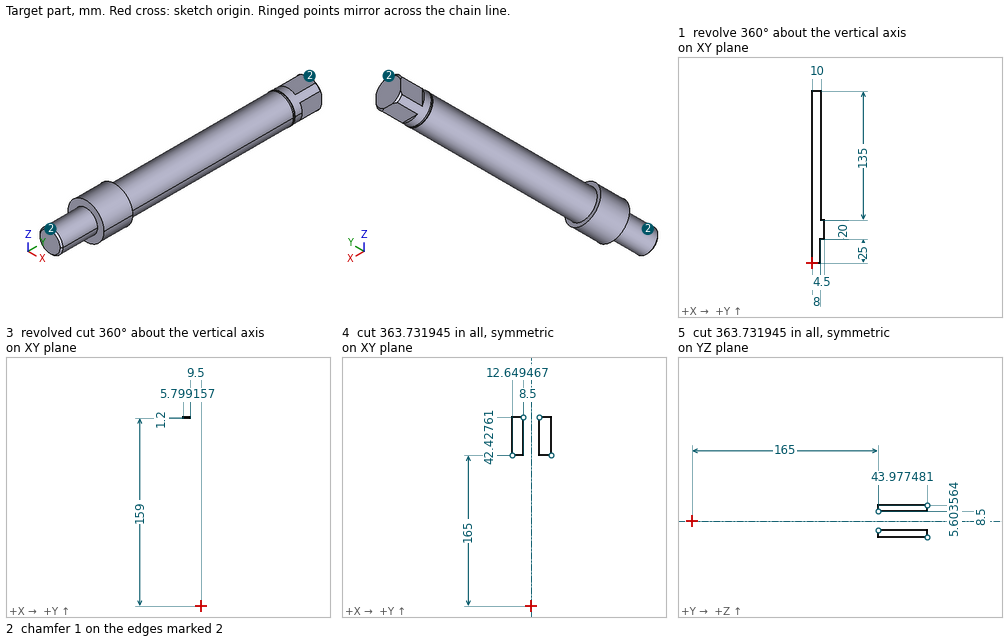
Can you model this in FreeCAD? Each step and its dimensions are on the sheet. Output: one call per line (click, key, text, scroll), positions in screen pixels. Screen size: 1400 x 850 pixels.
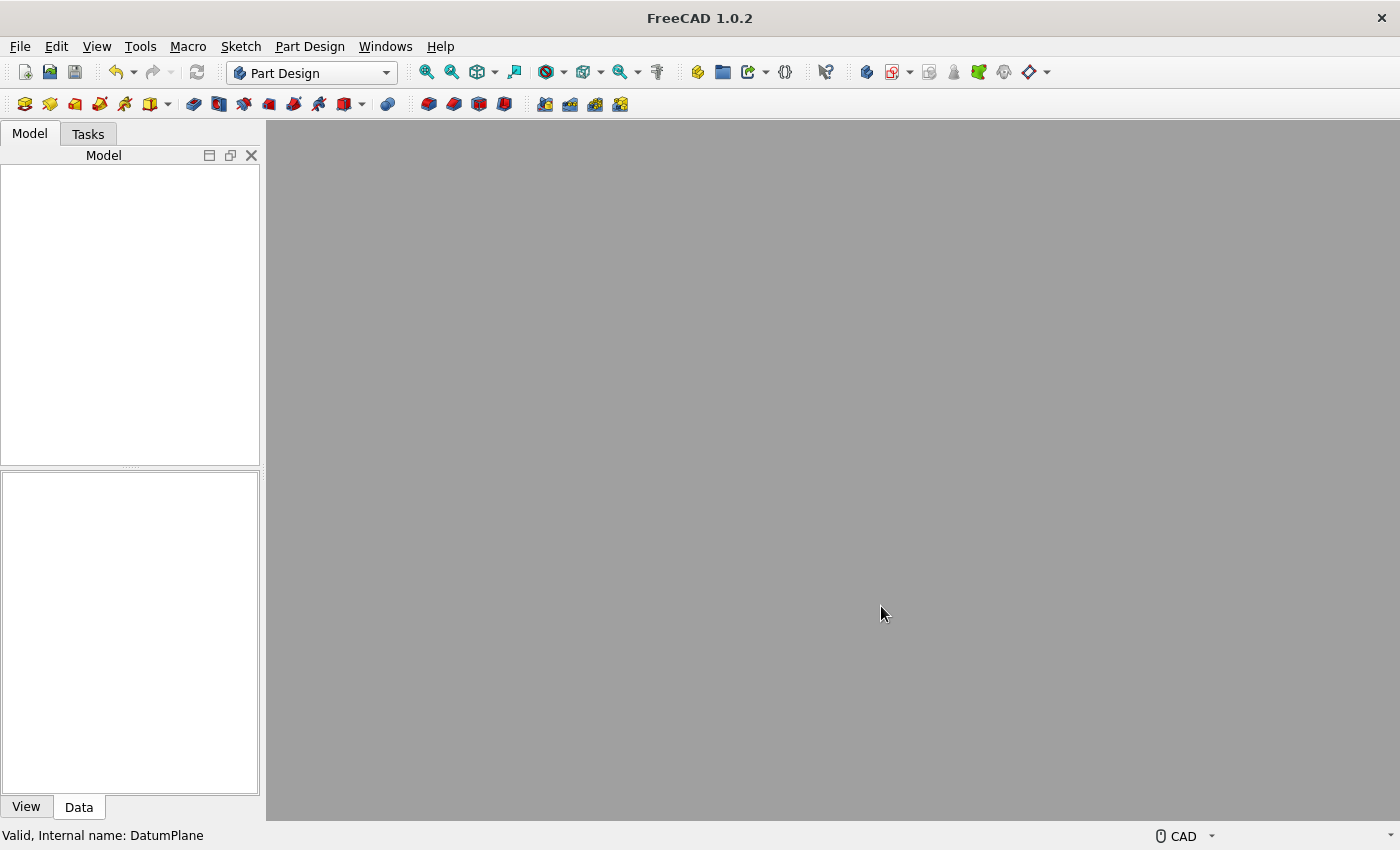
key(ctrl+n)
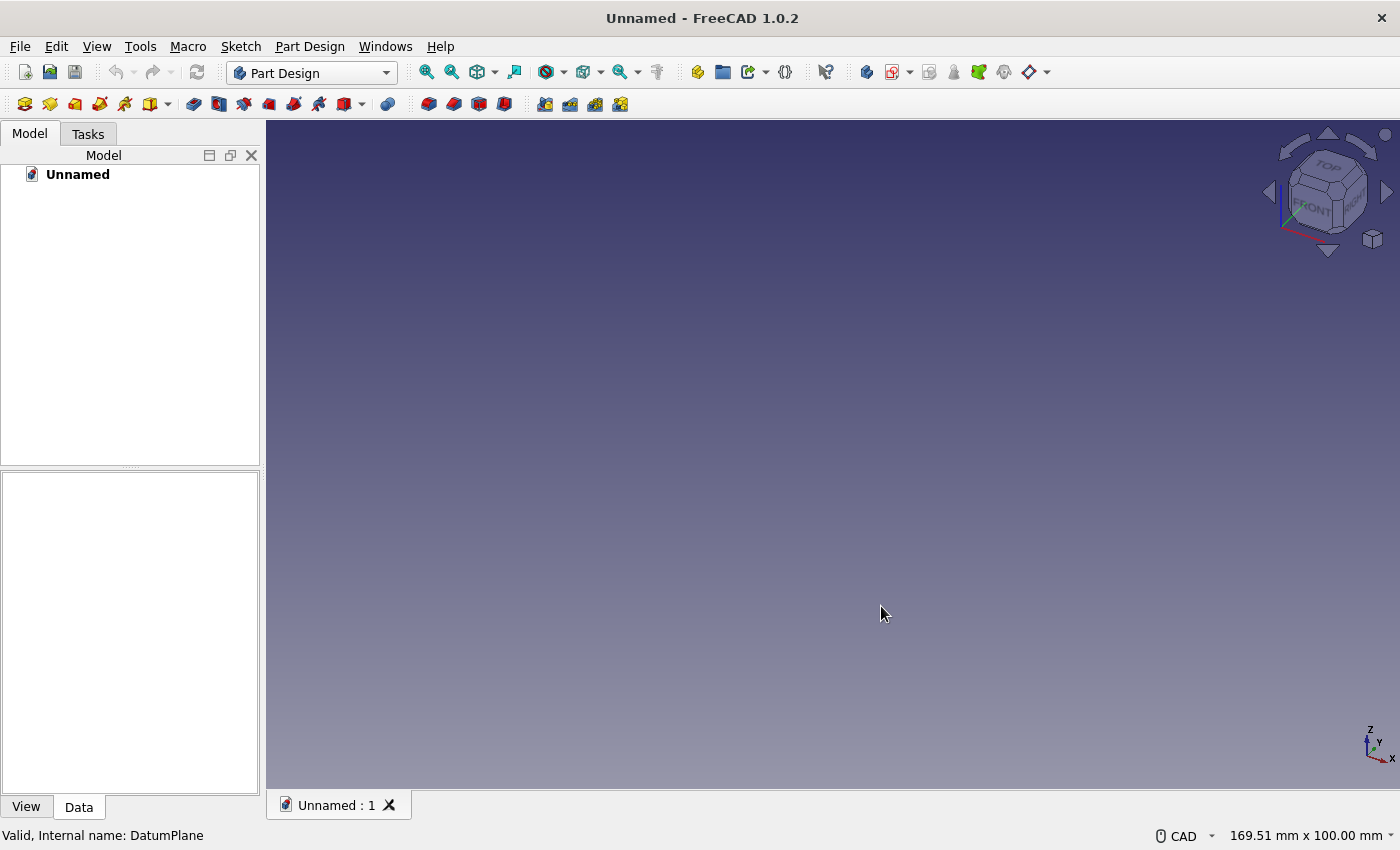
click(892, 72)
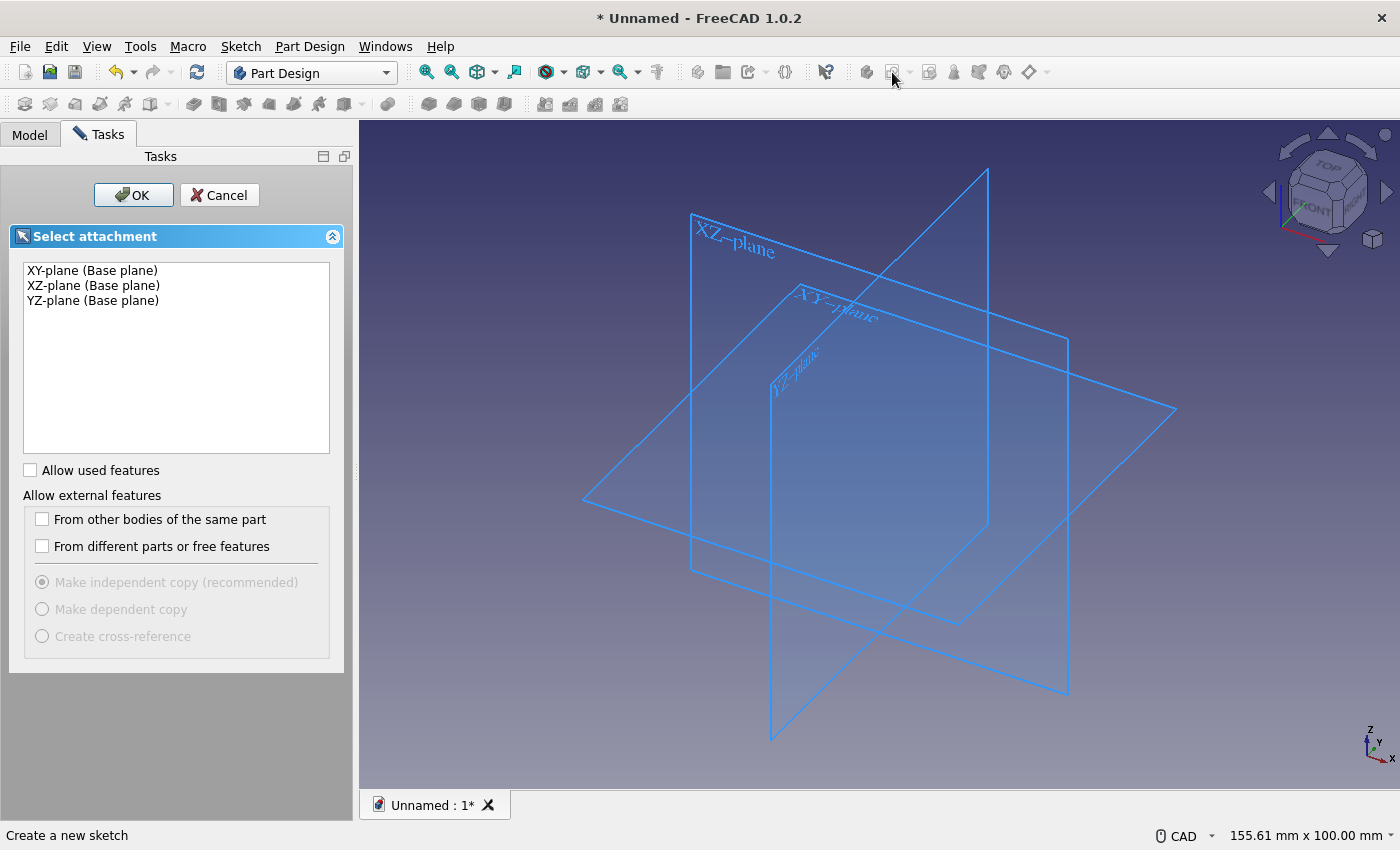
click(84, 270)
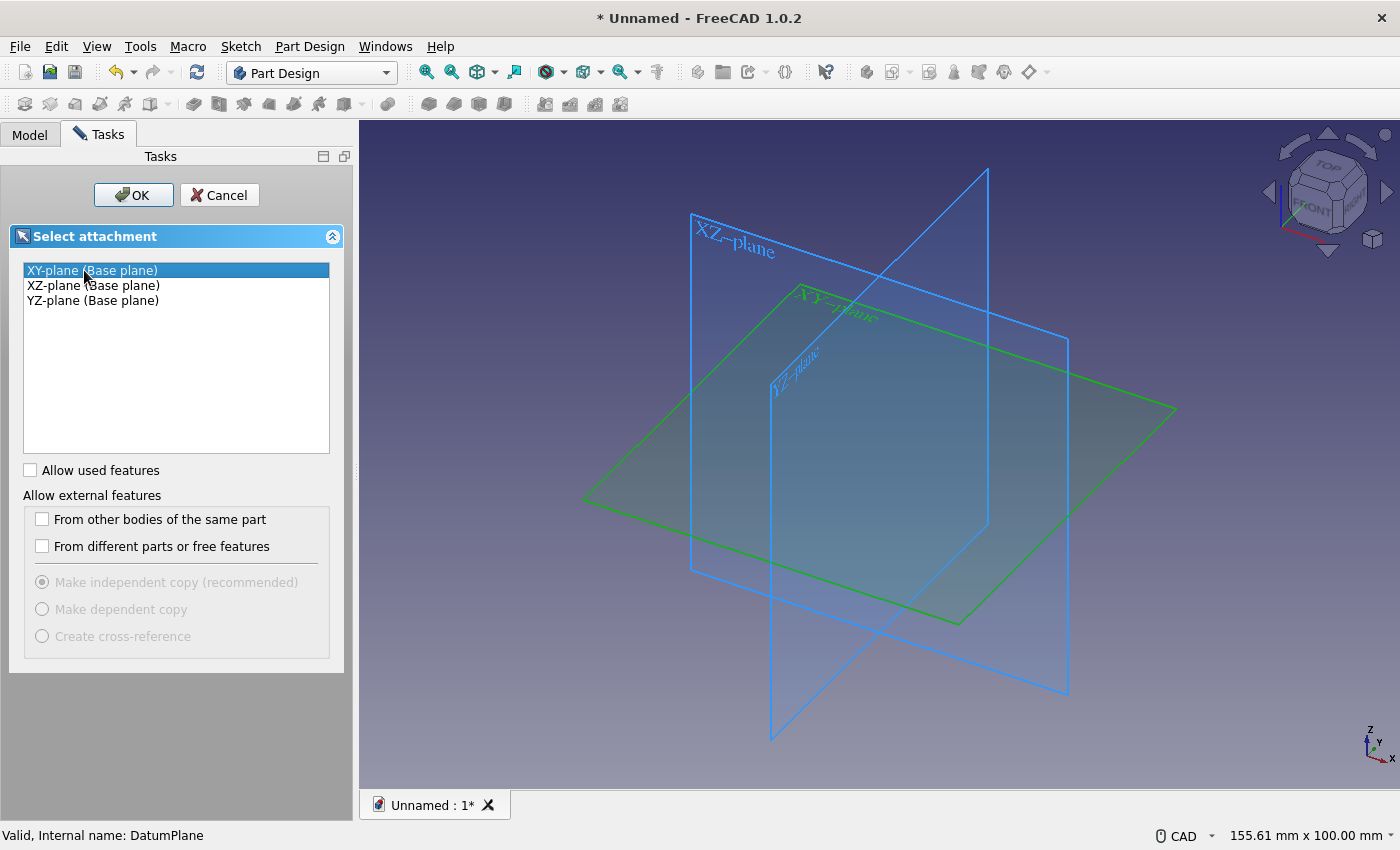
click(134, 195)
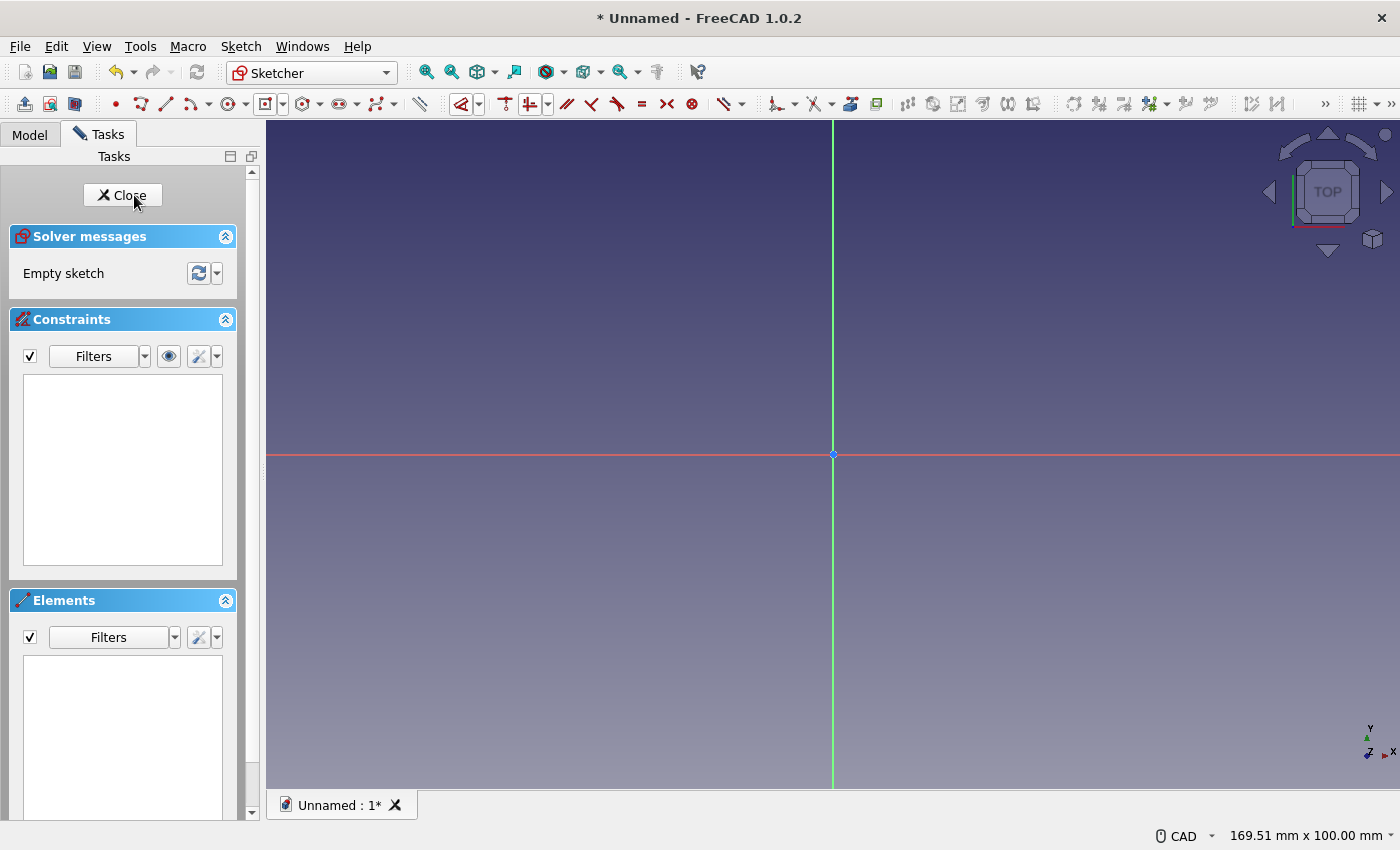
scroll(700, 761, down, 5)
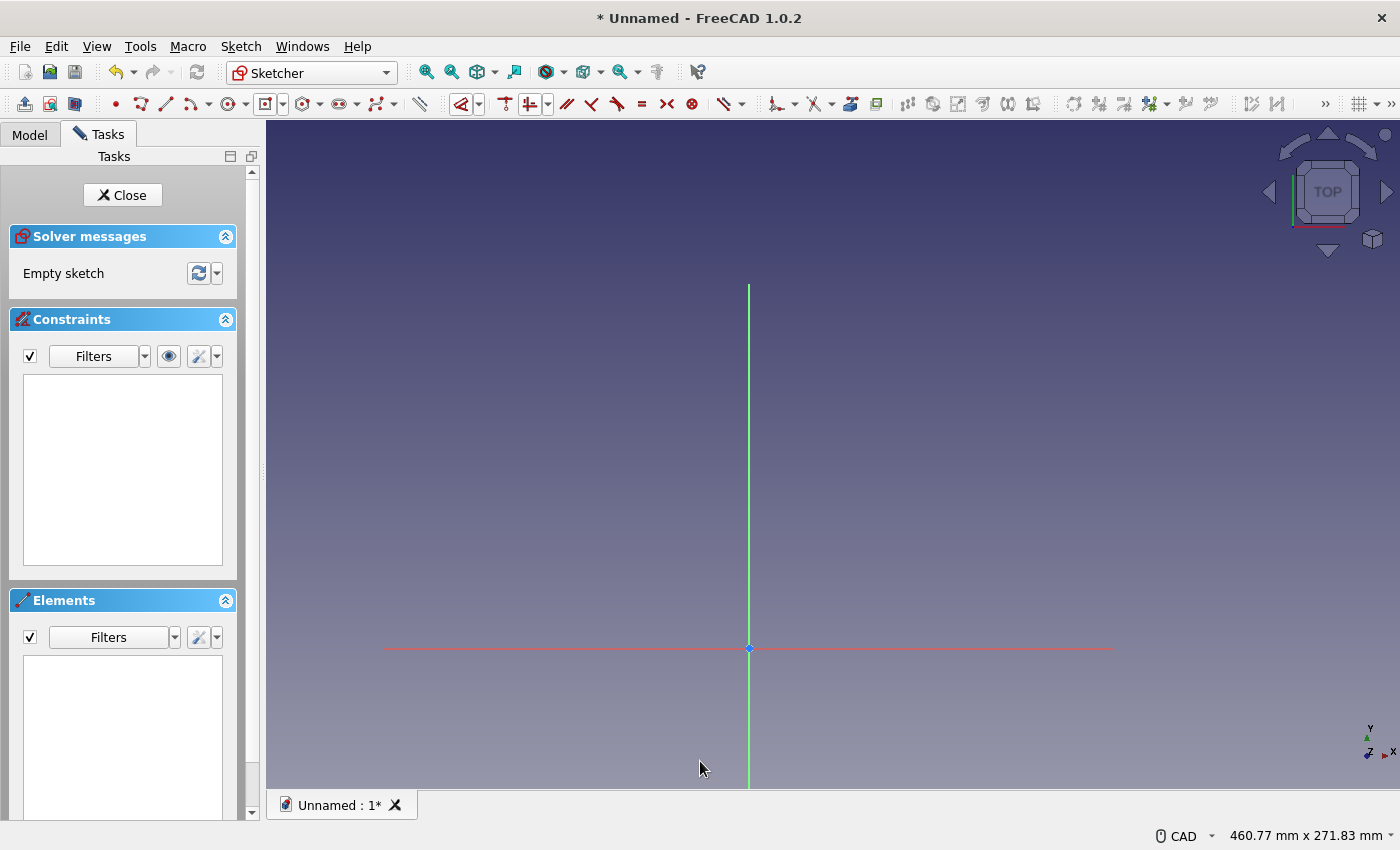
key(g)
key(m)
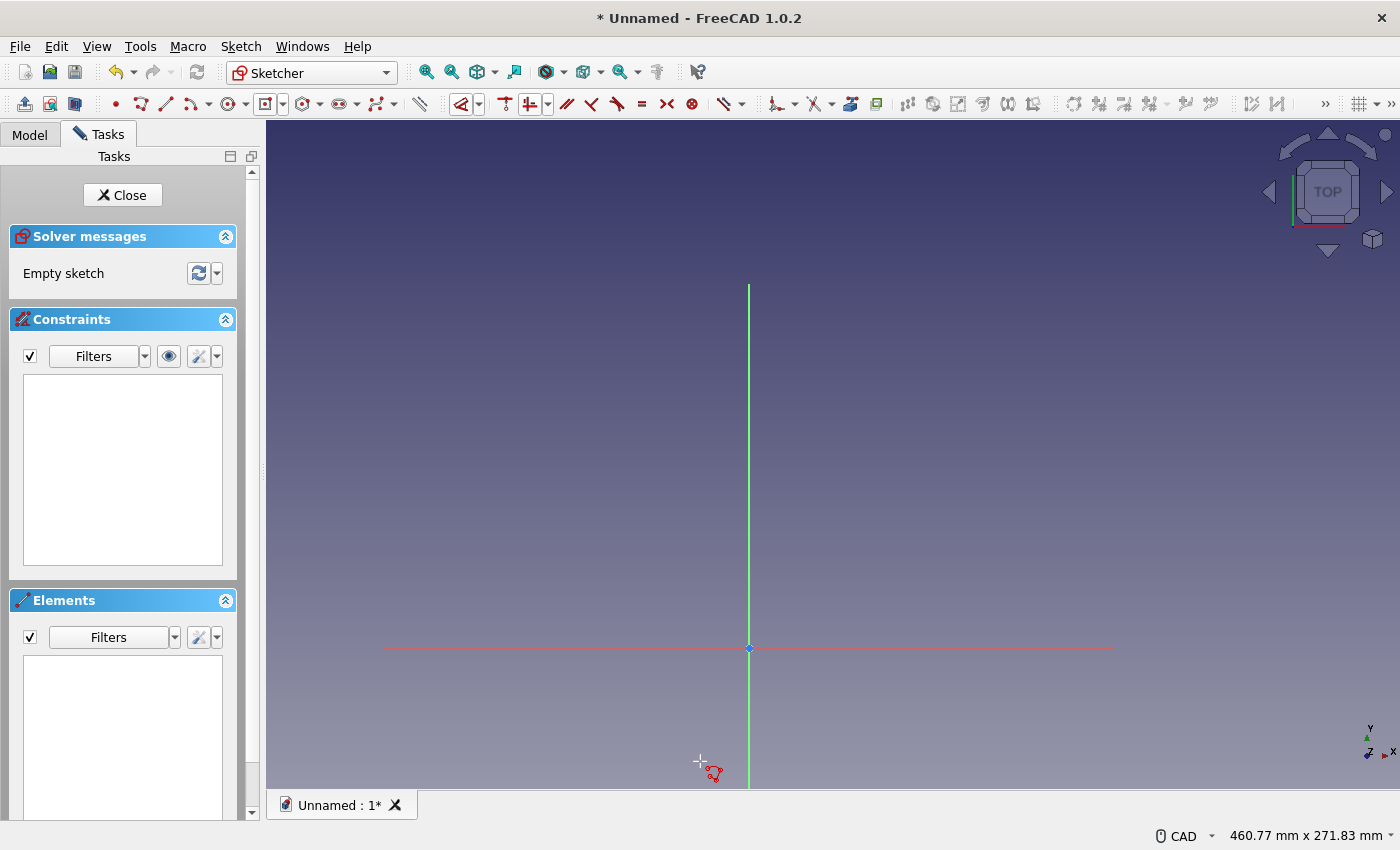
click(749, 649)
click(769, 640)
click(769, 587)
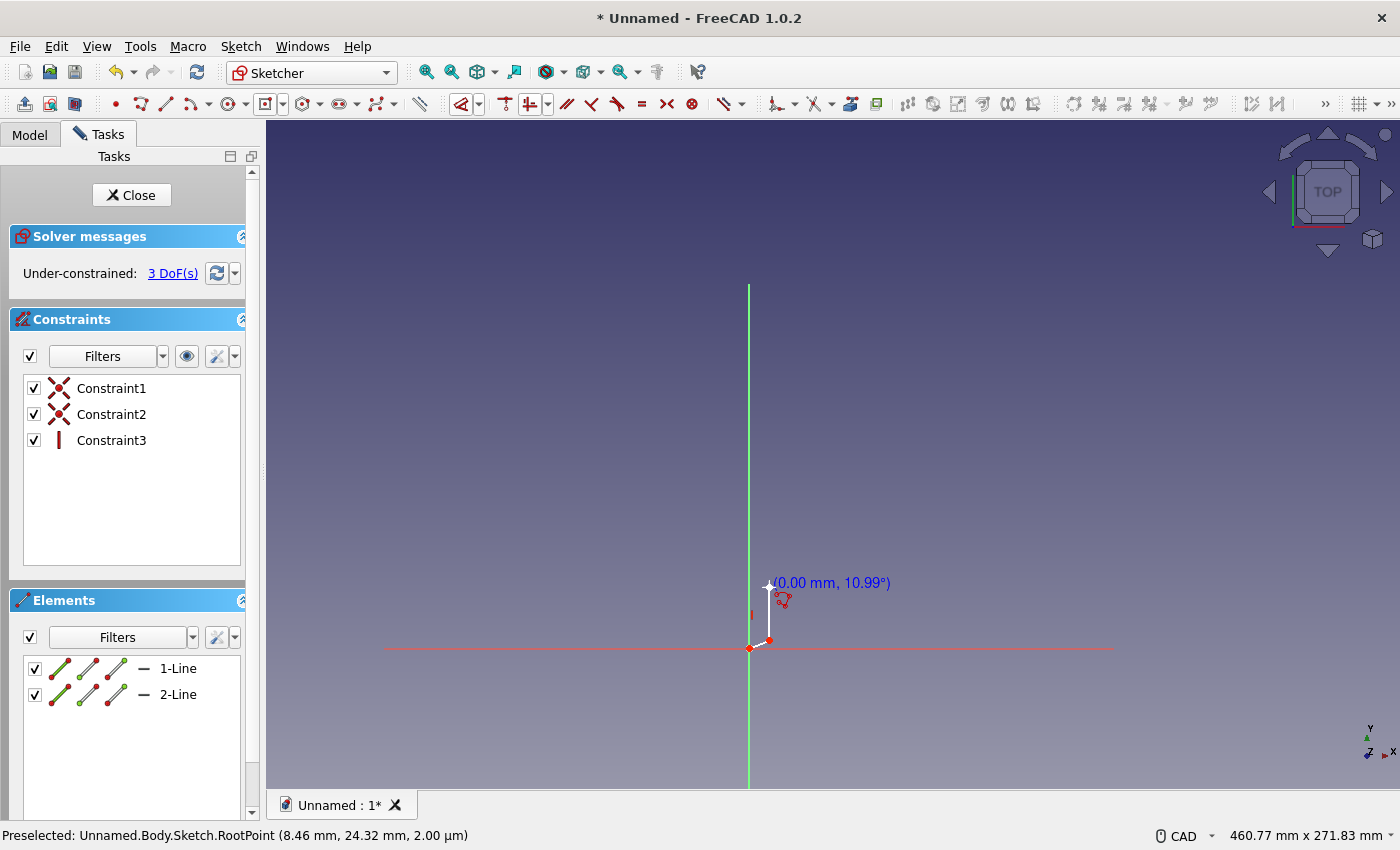
scroll(780, 587, up, 2)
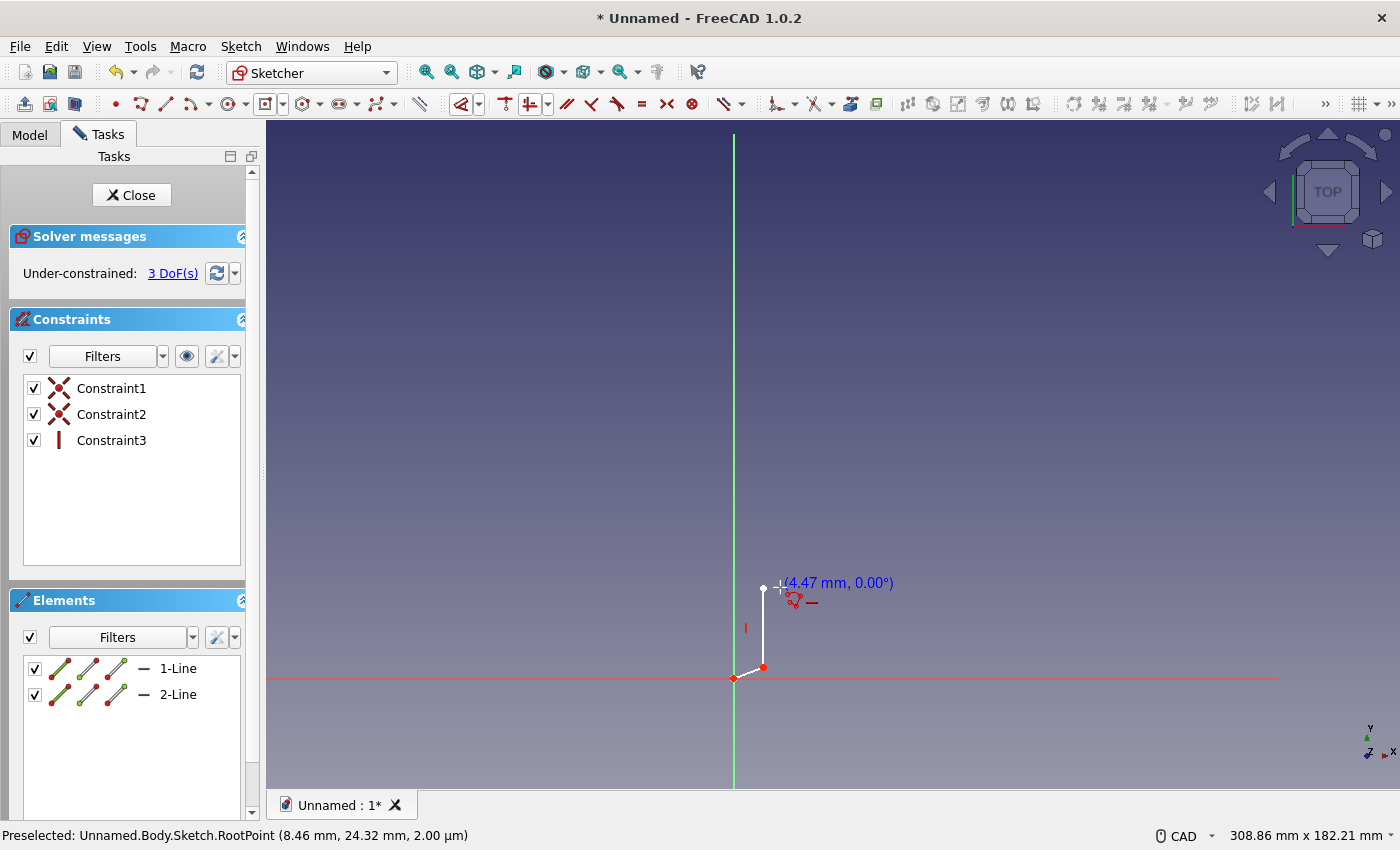
click(780, 587)
click(780, 514)